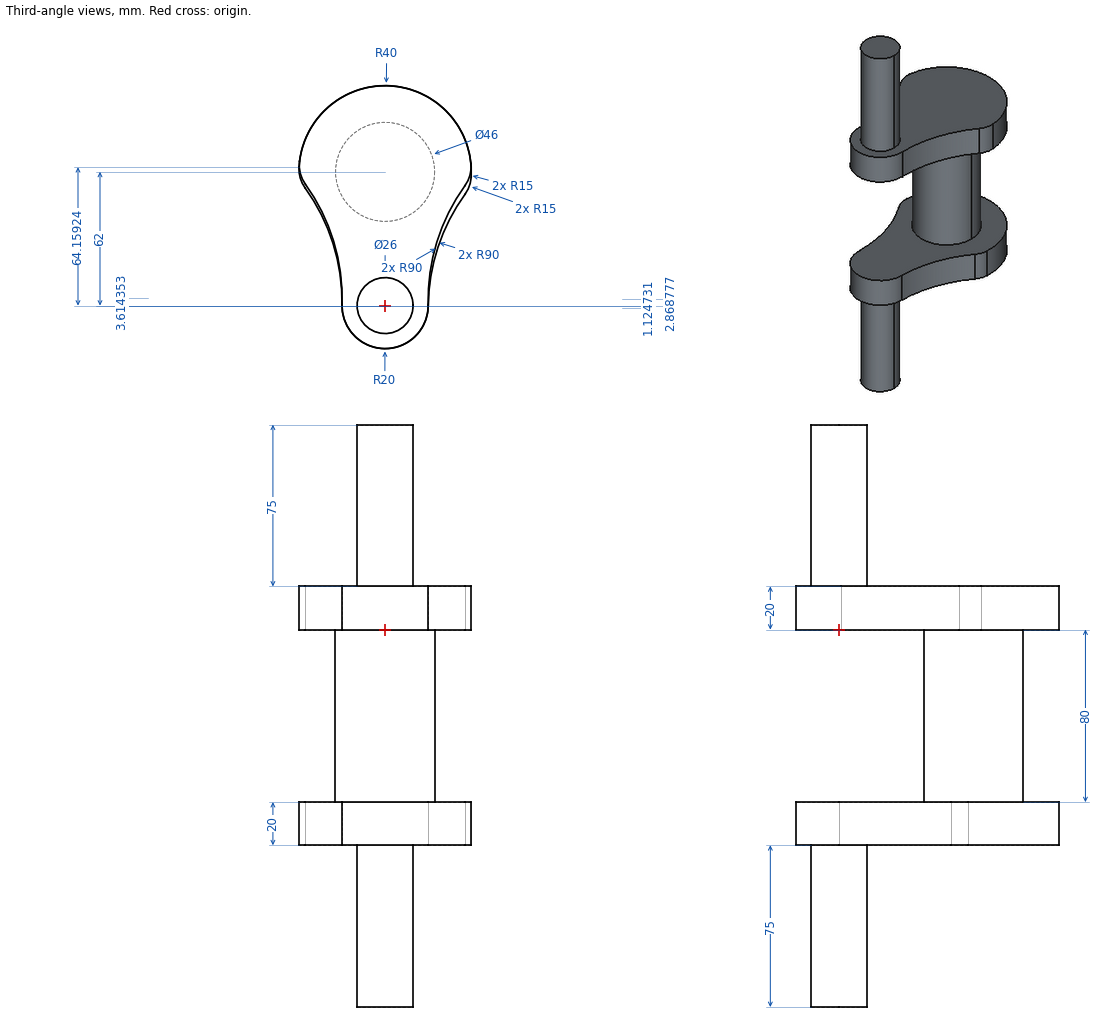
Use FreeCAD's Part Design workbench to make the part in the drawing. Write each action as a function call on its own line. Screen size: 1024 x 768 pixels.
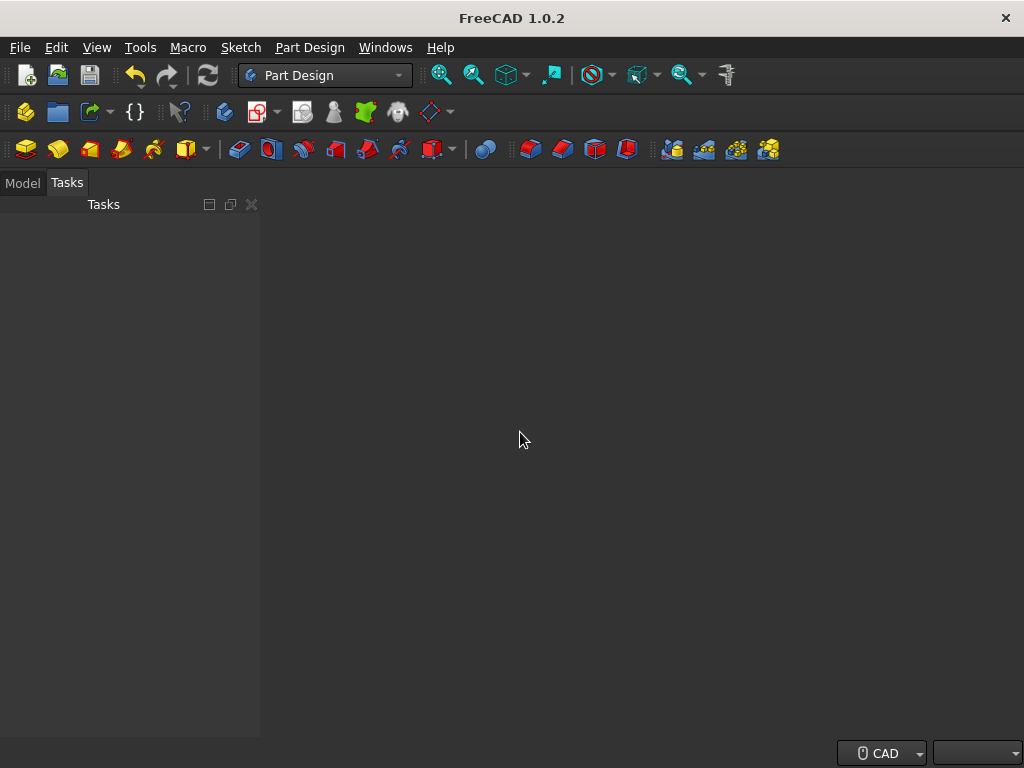
click(26, 76)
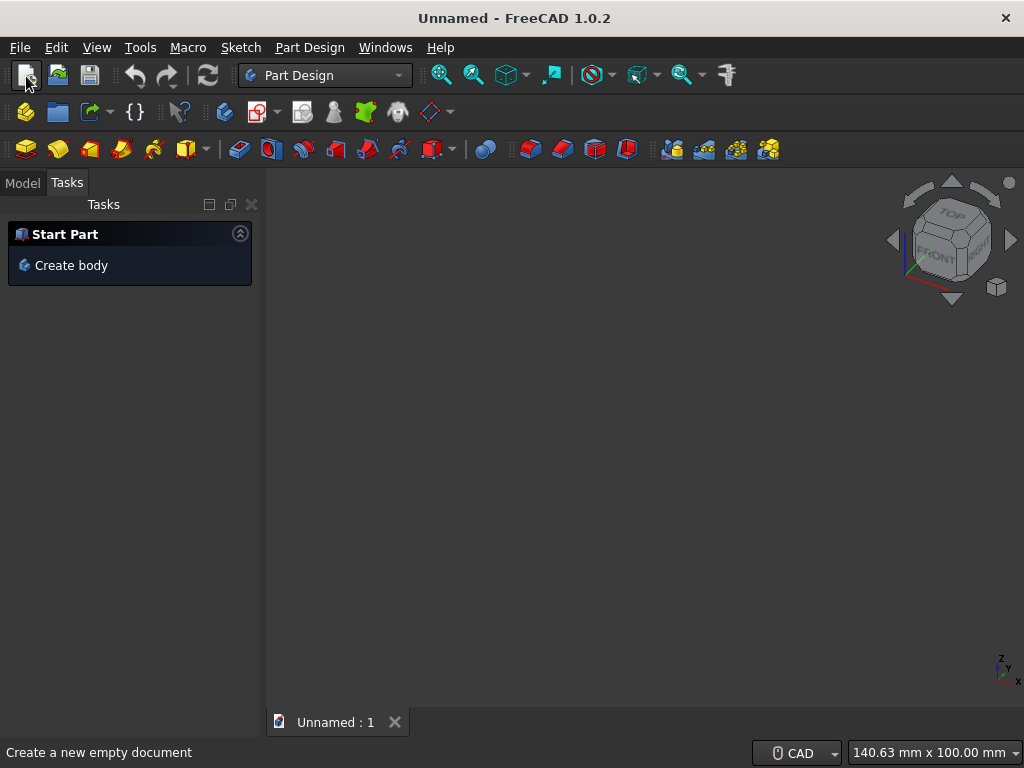
click(258, 112)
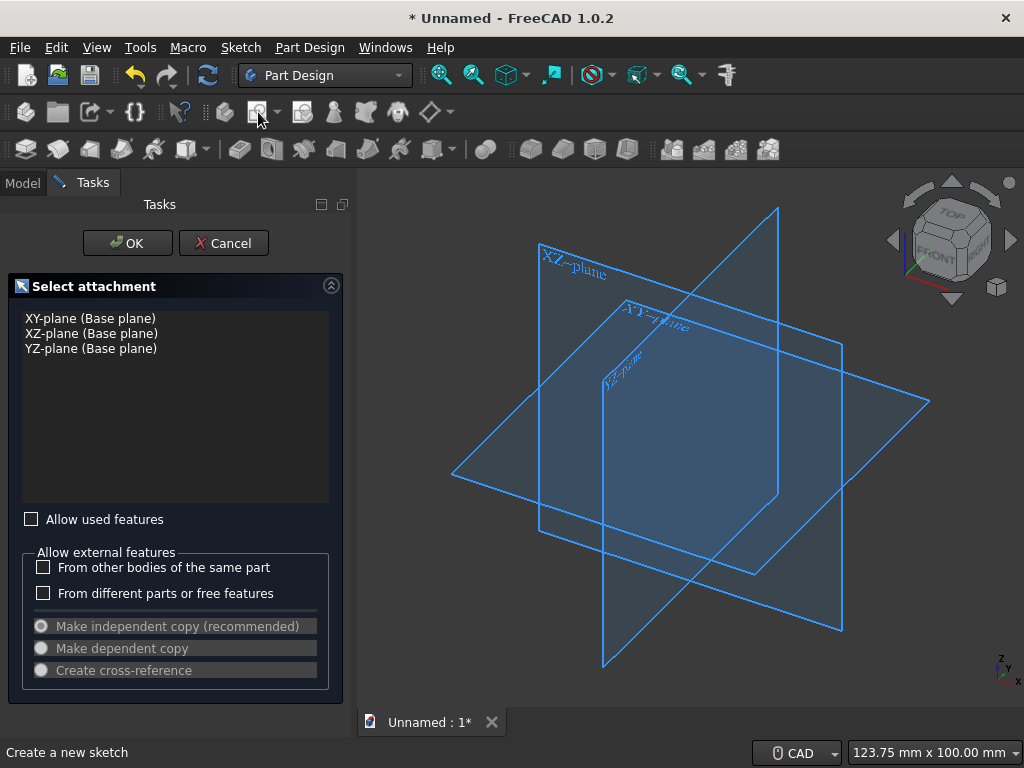
click(82, 318)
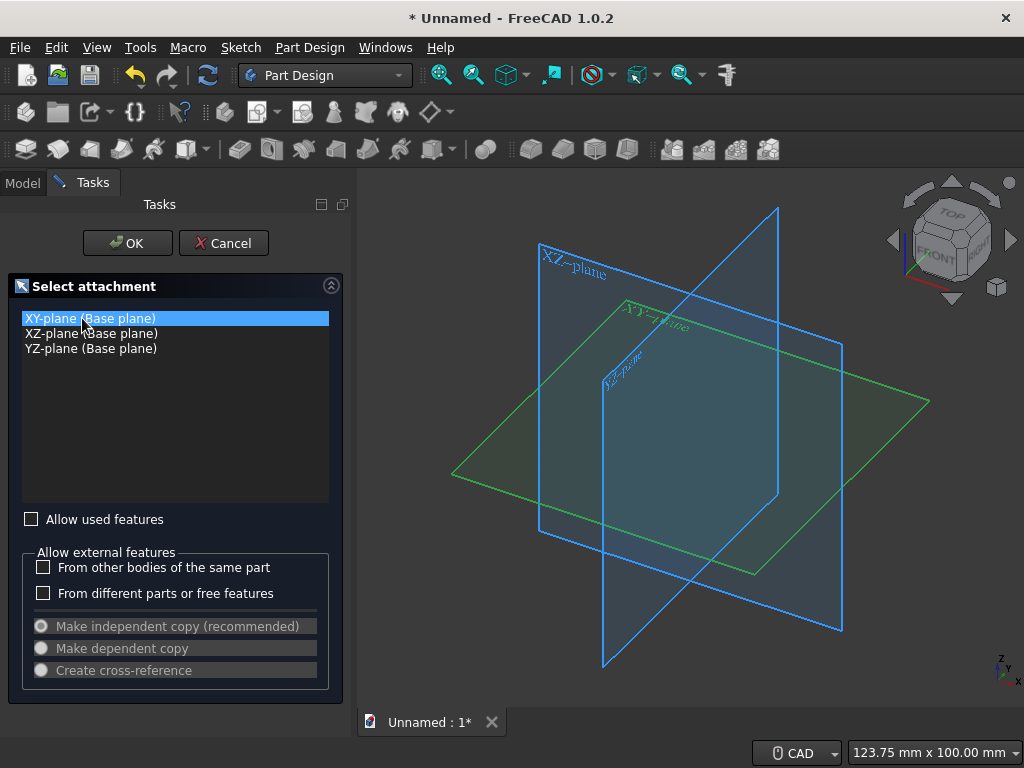
click(128, 243)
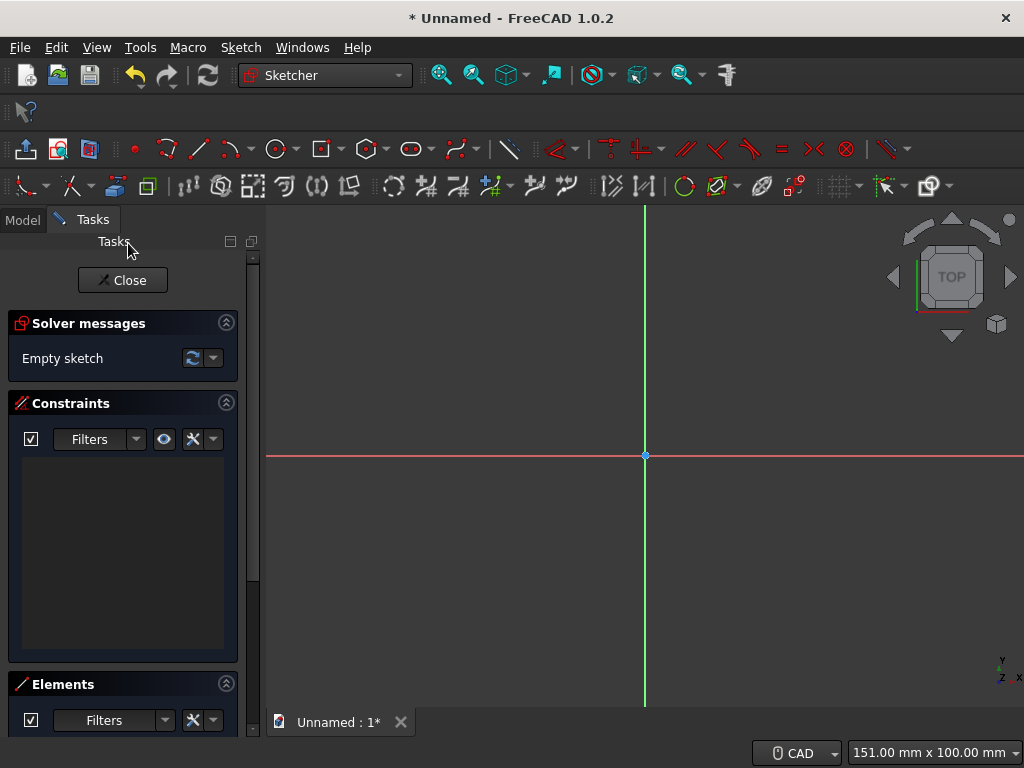
scroll(493, 679, down, 3)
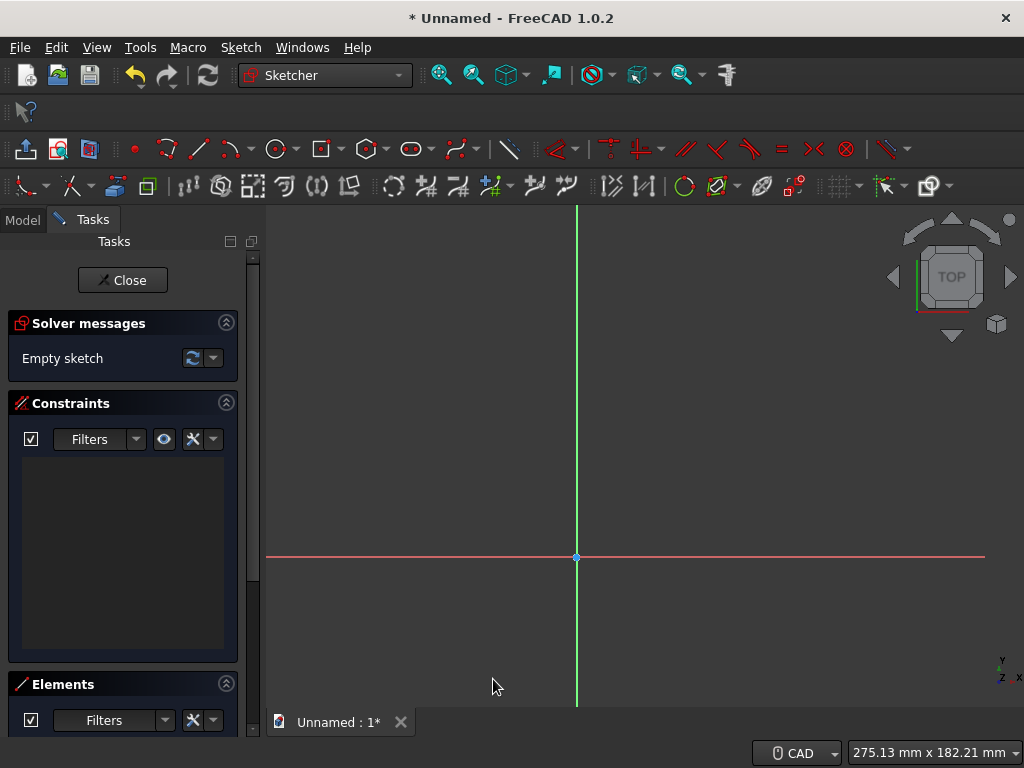
key(g)
key(3)
key(a)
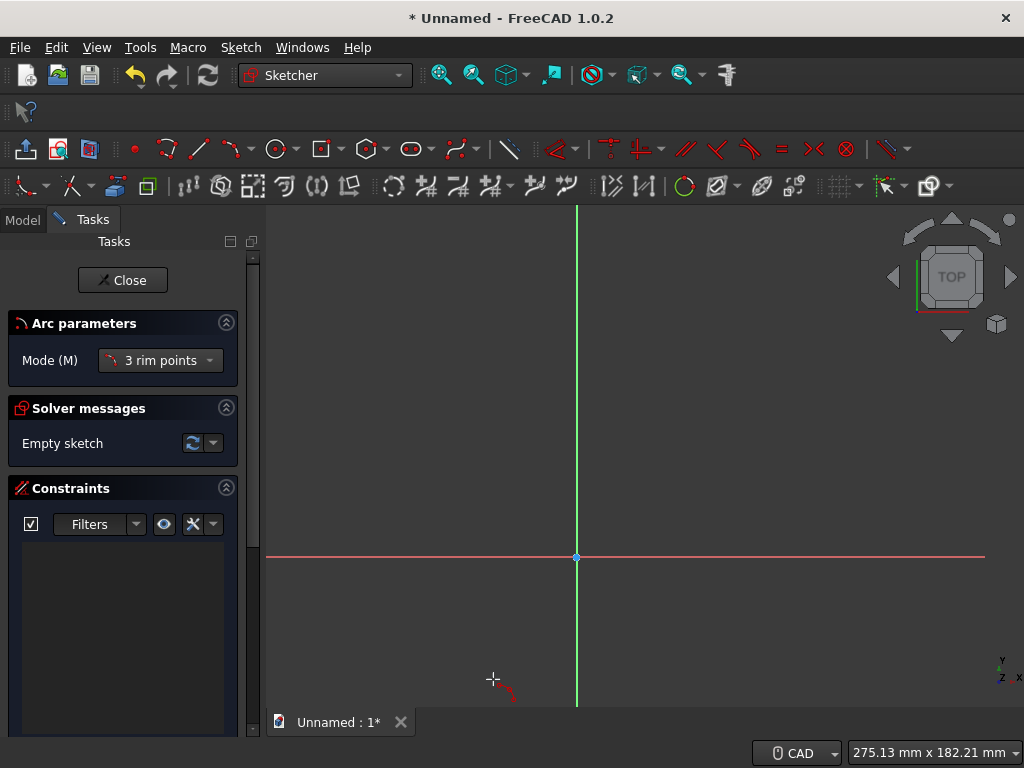
scroll(632, 556, up, 13)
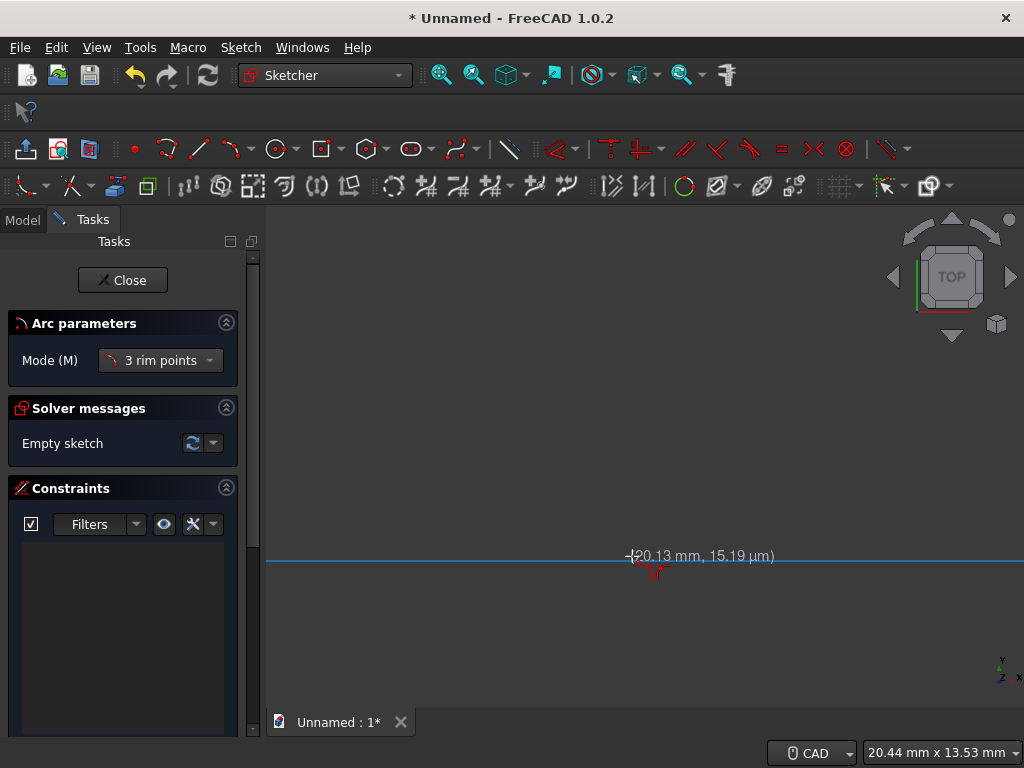
click(621, 542)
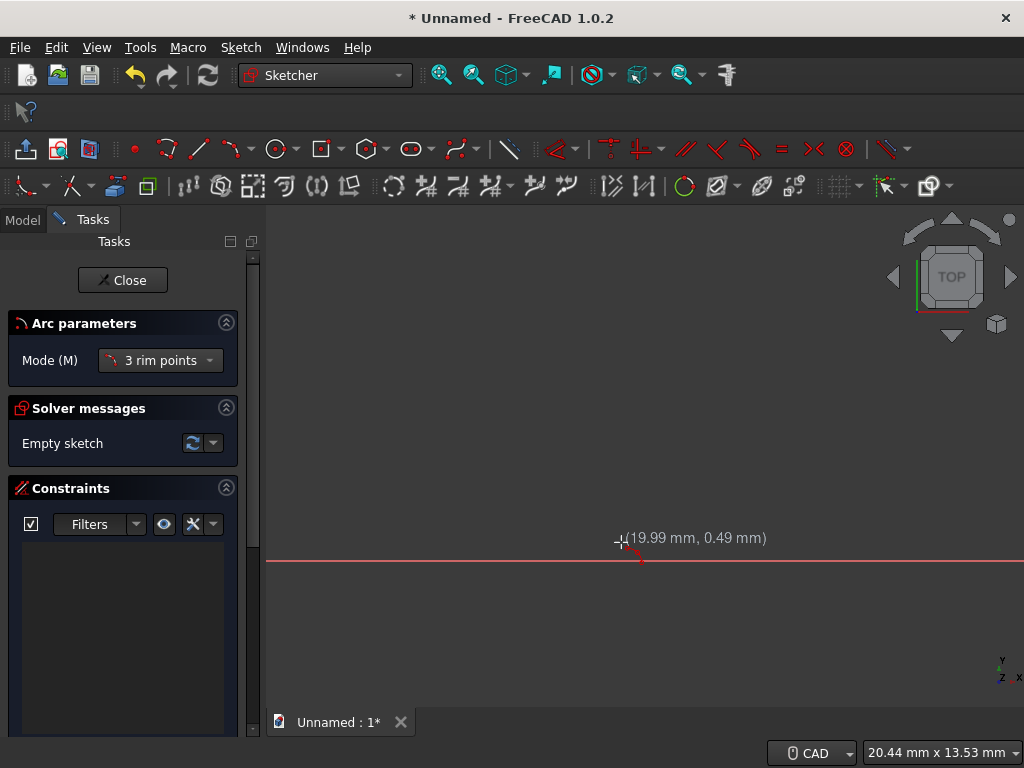
scroll(632, 570, down, 13)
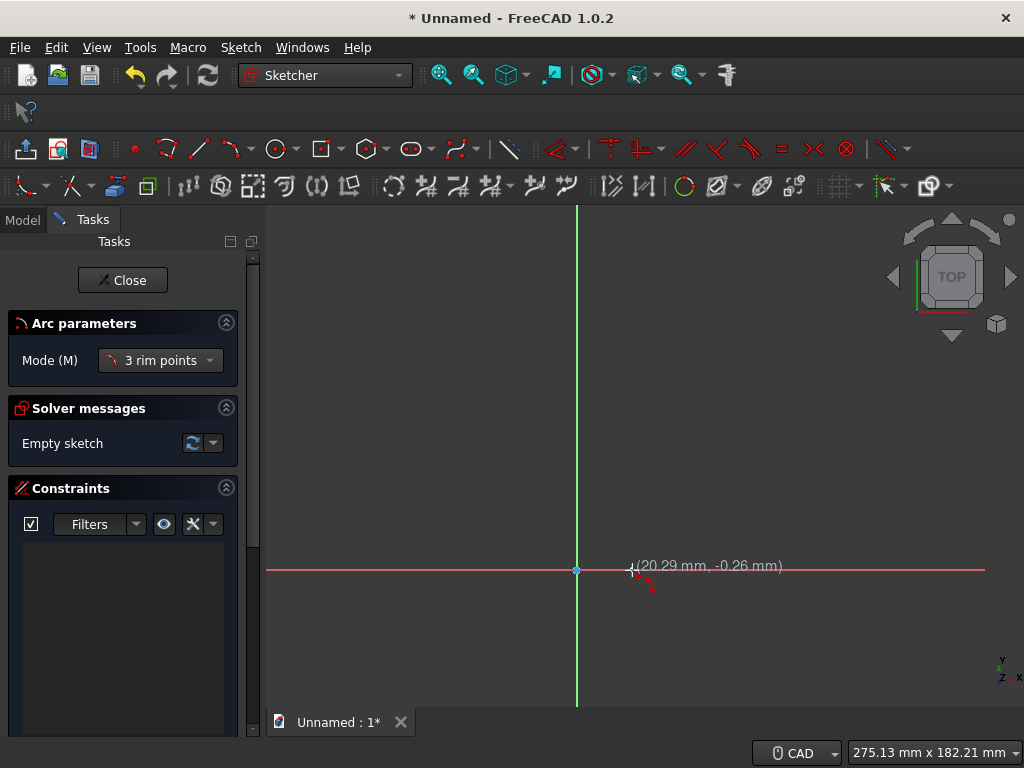
click(679, 417)
click(643, 489)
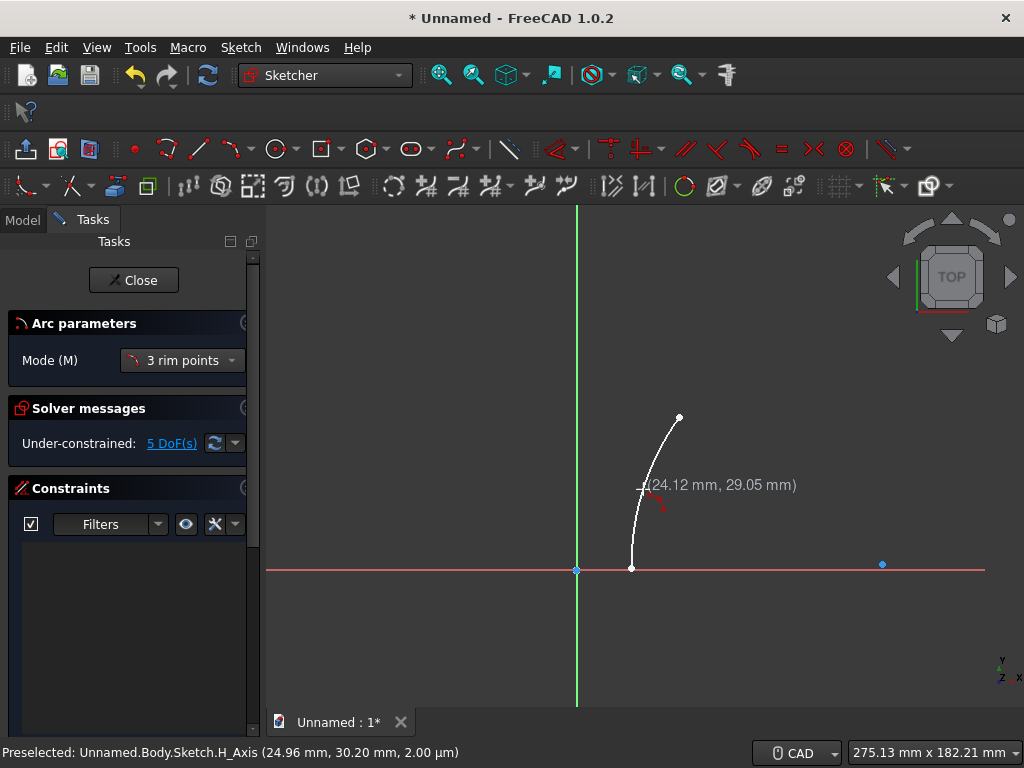
click(679, 418)
click(686, 389)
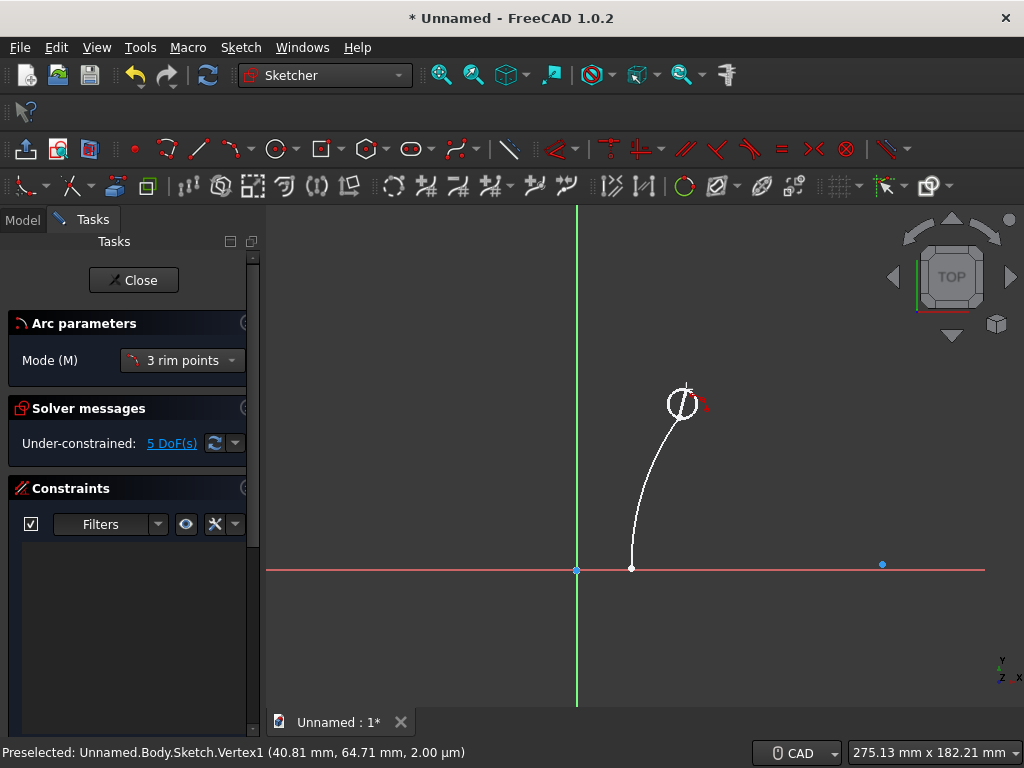
scroll(685, 403, up, 9)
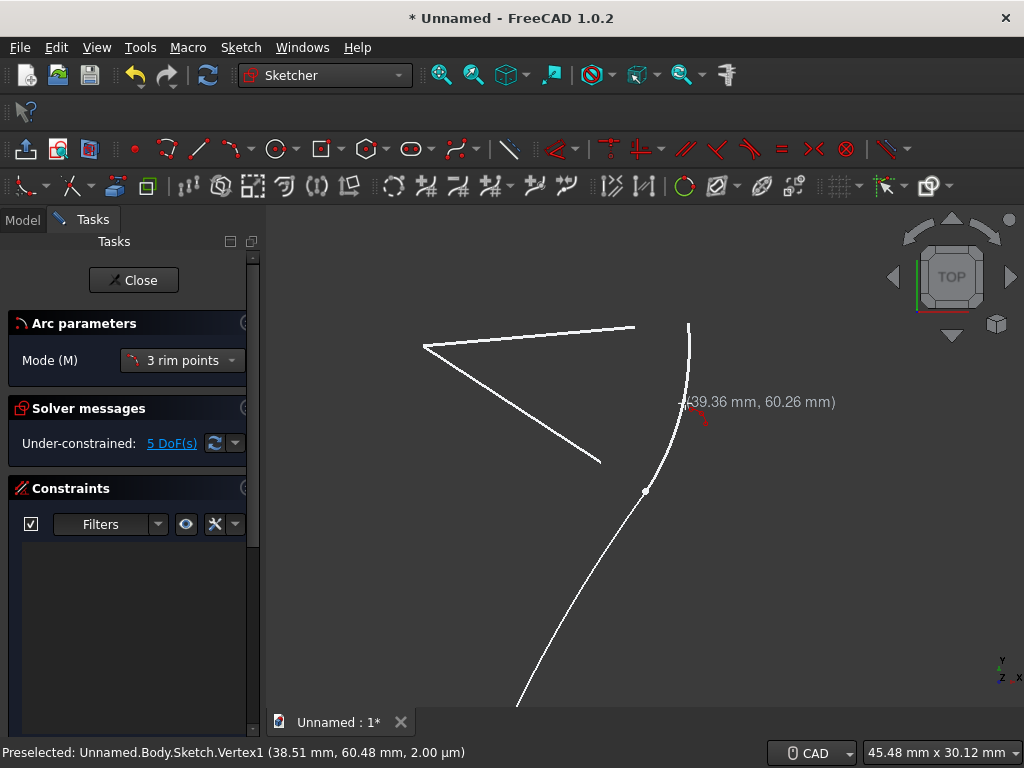
click(682, 403)